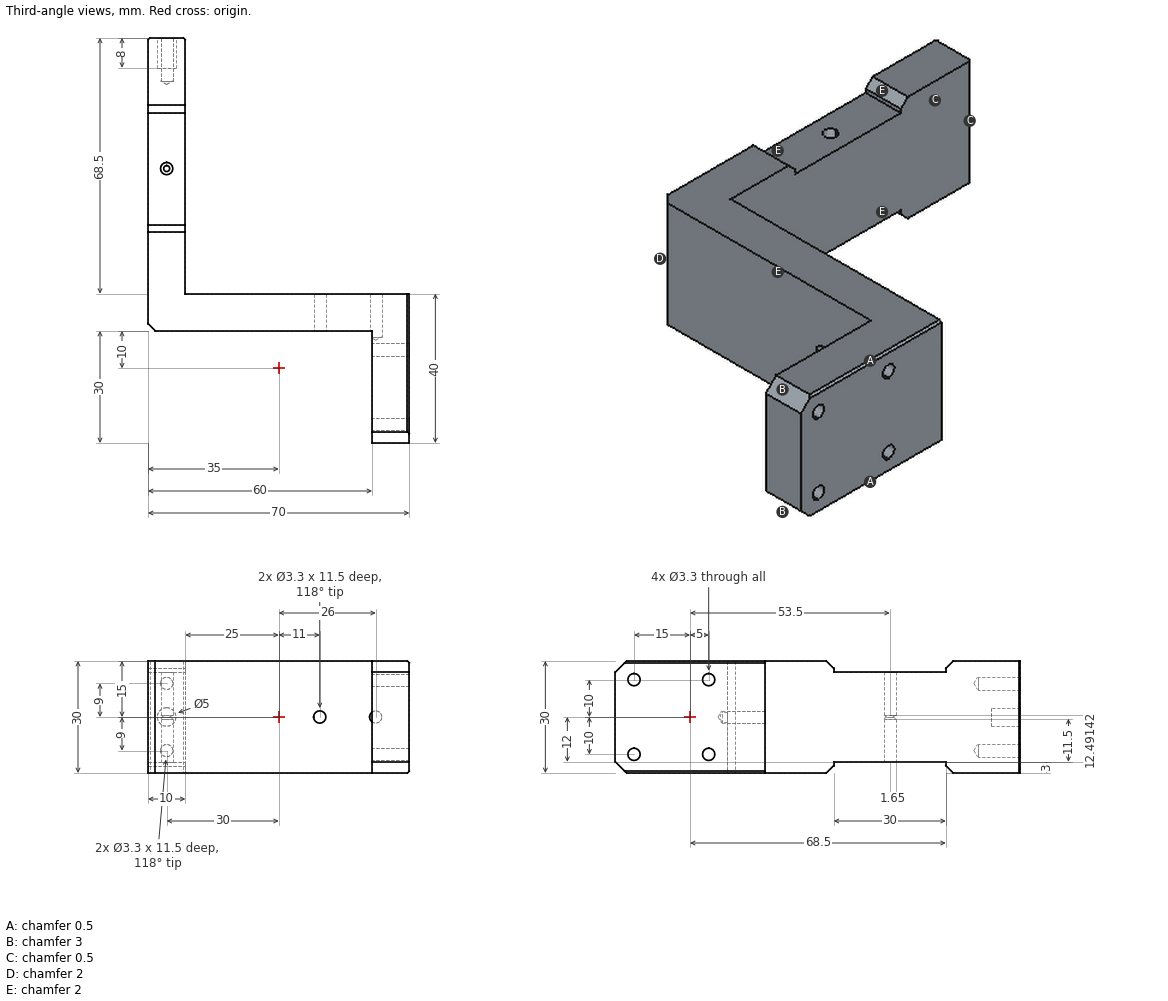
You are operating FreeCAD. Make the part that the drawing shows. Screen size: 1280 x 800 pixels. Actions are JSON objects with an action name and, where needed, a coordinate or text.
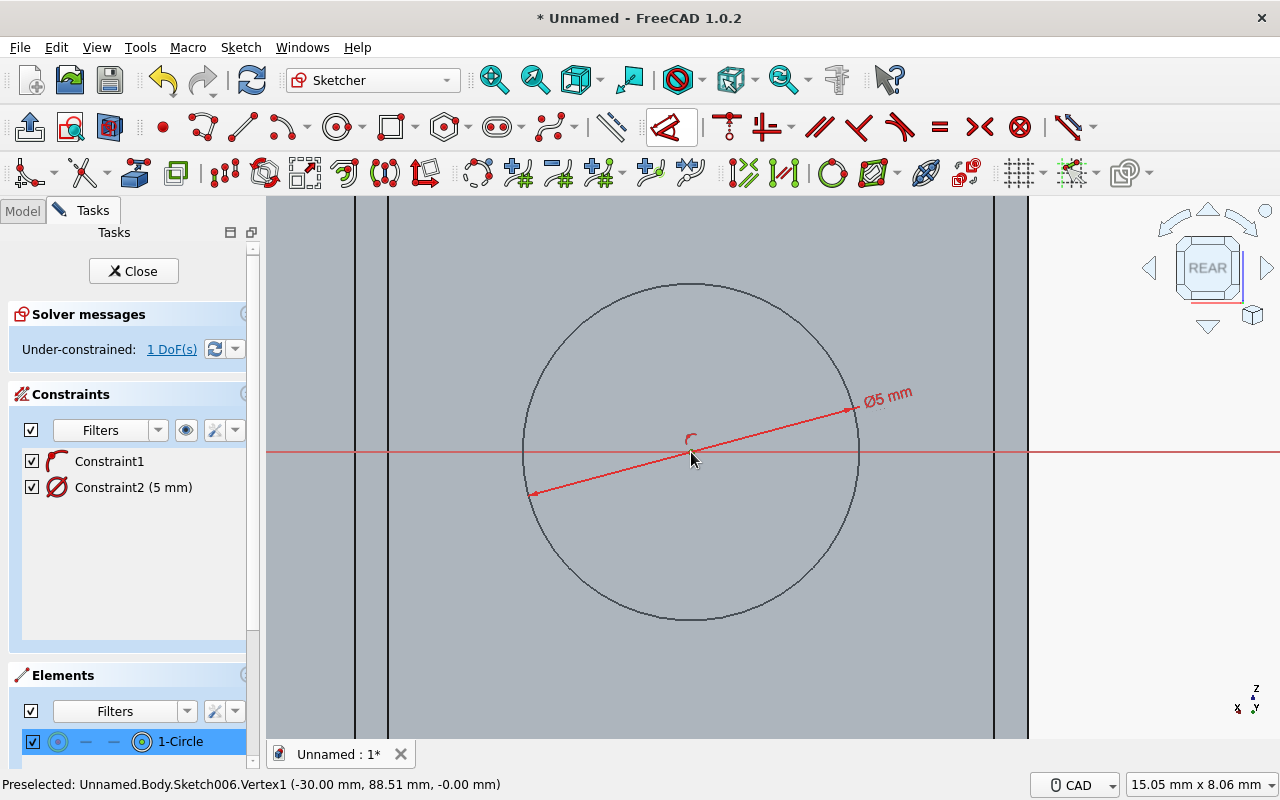
{"action": "left_click", "coordinate": [692, 128]}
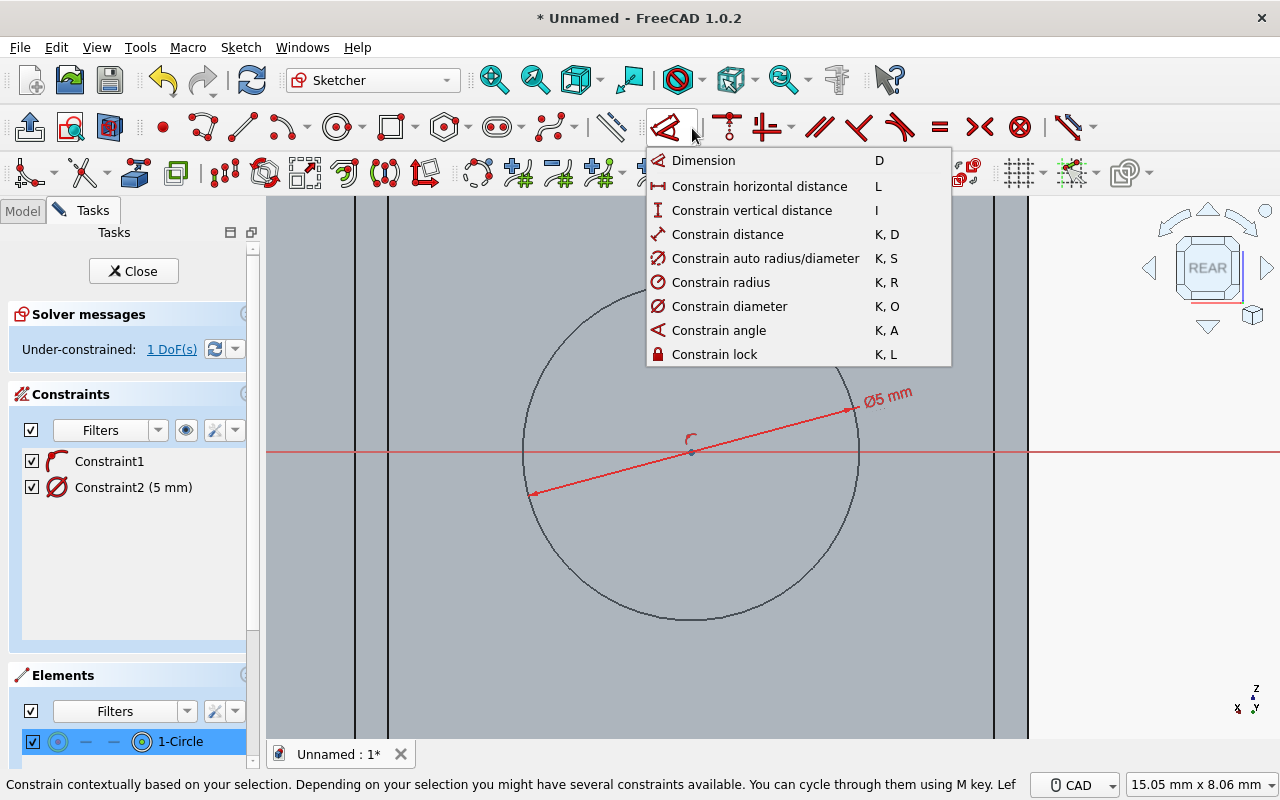
{"action": "left_click", "coordinate": [799, 186]}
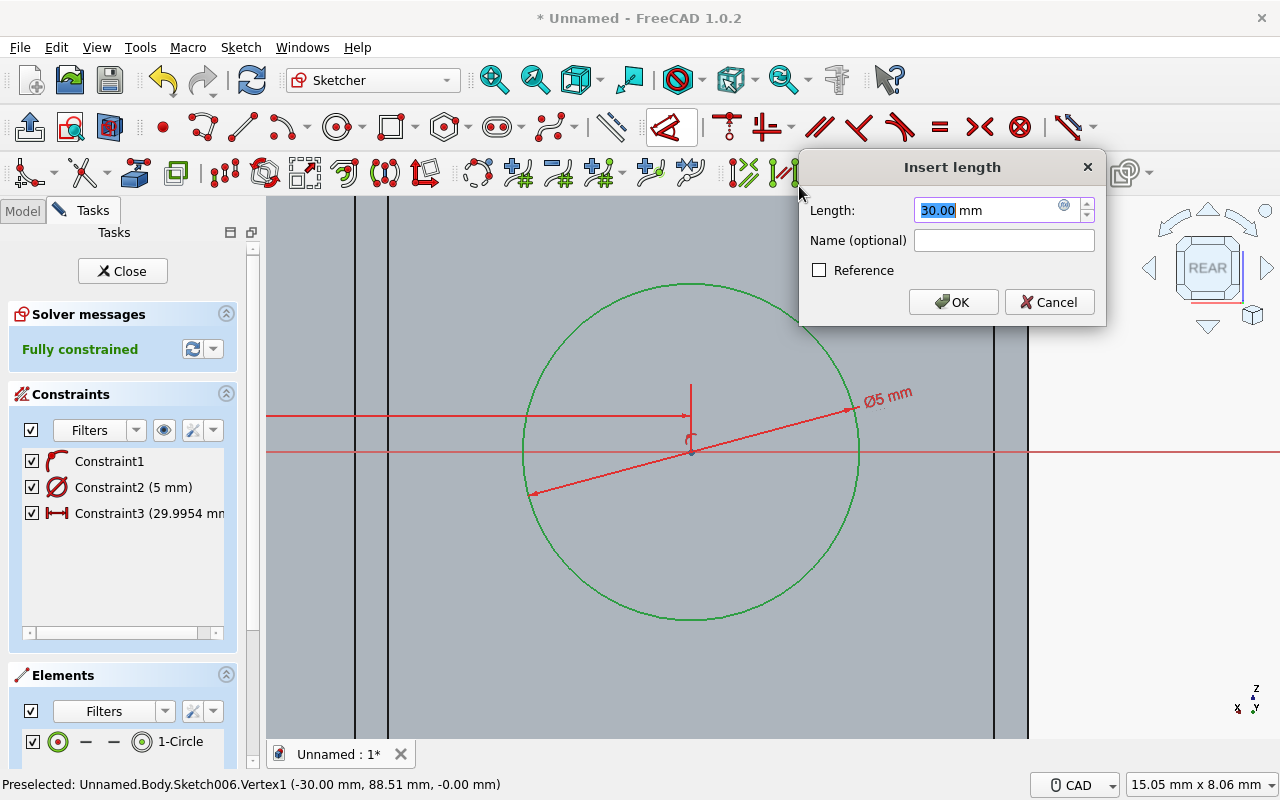
{"action": "type", "text": "30"}
{"action": "key", "text": "Return"}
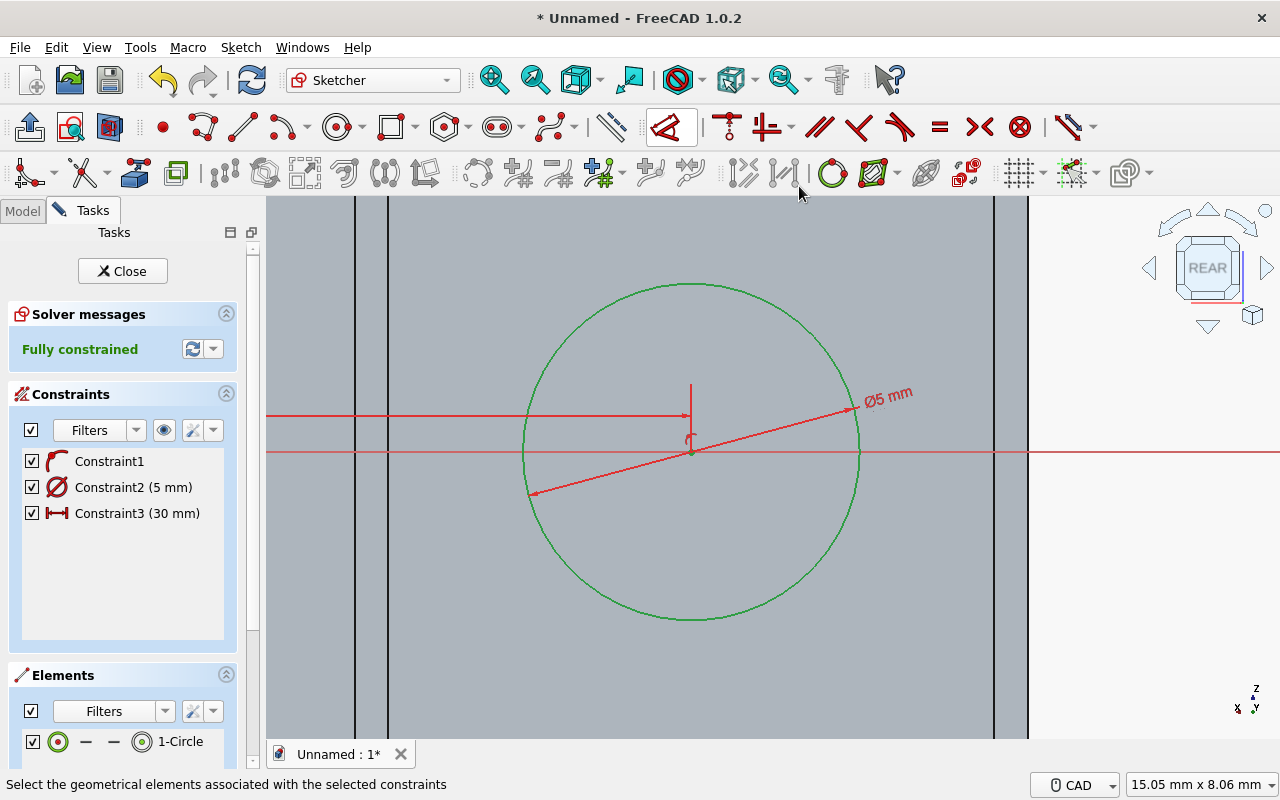
{"action": "left_click", "coordinate": [123, 271]}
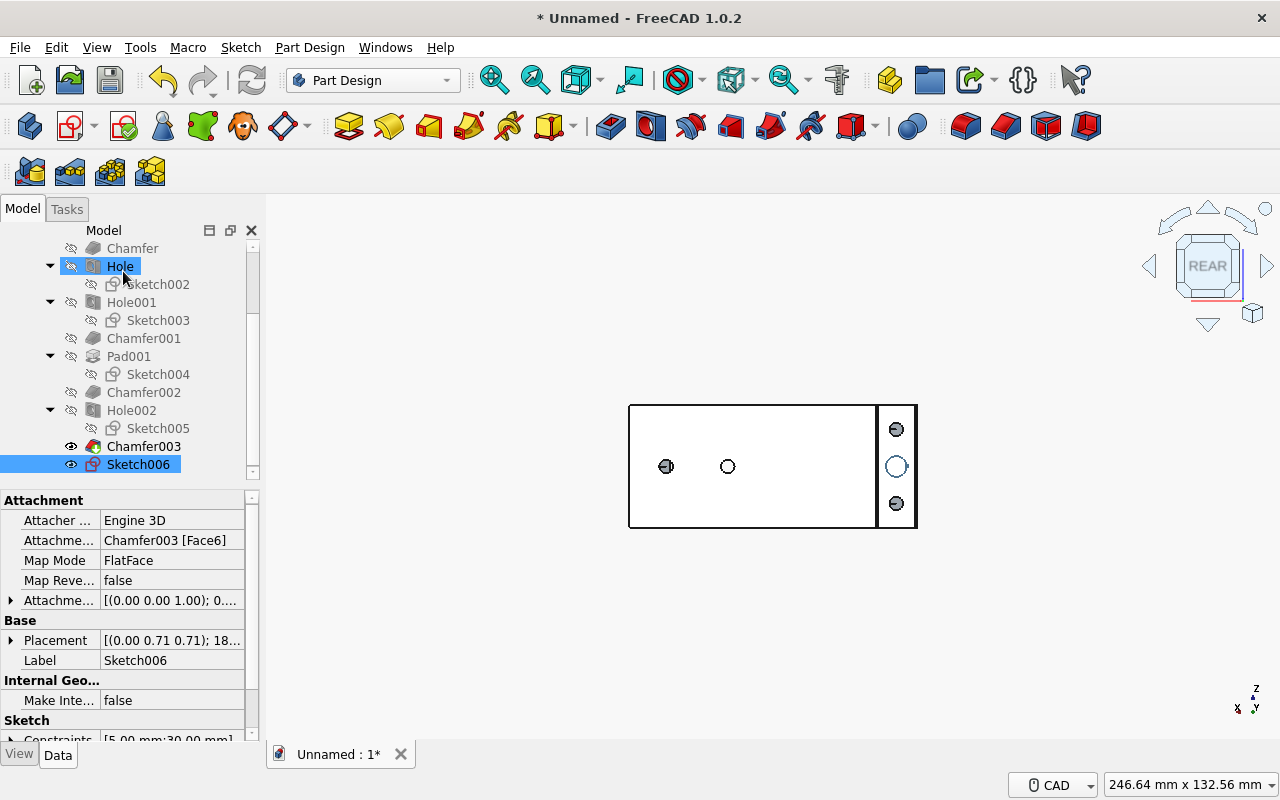
{"action": "left_click", "coordinate": [612, 126]}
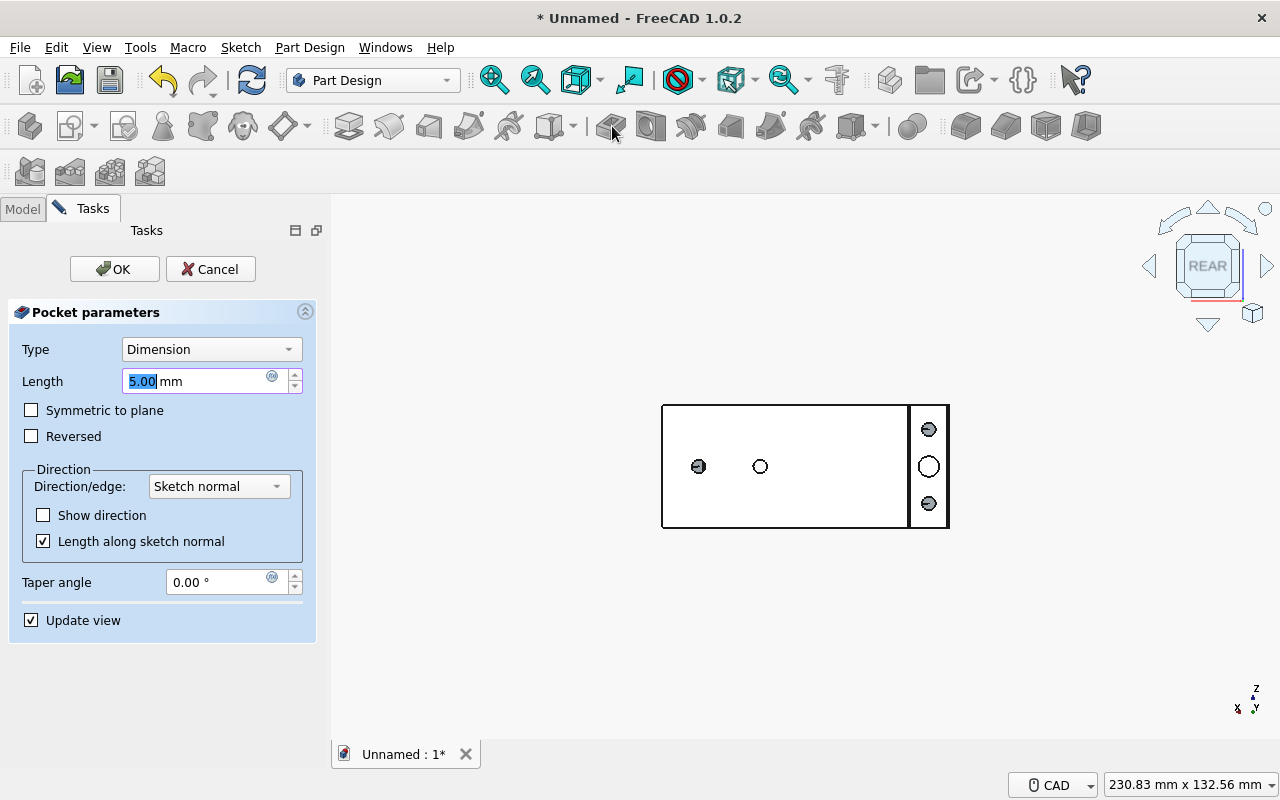
{"action": "type", "text": "8"}
{"action": "key", "text": "Tab"}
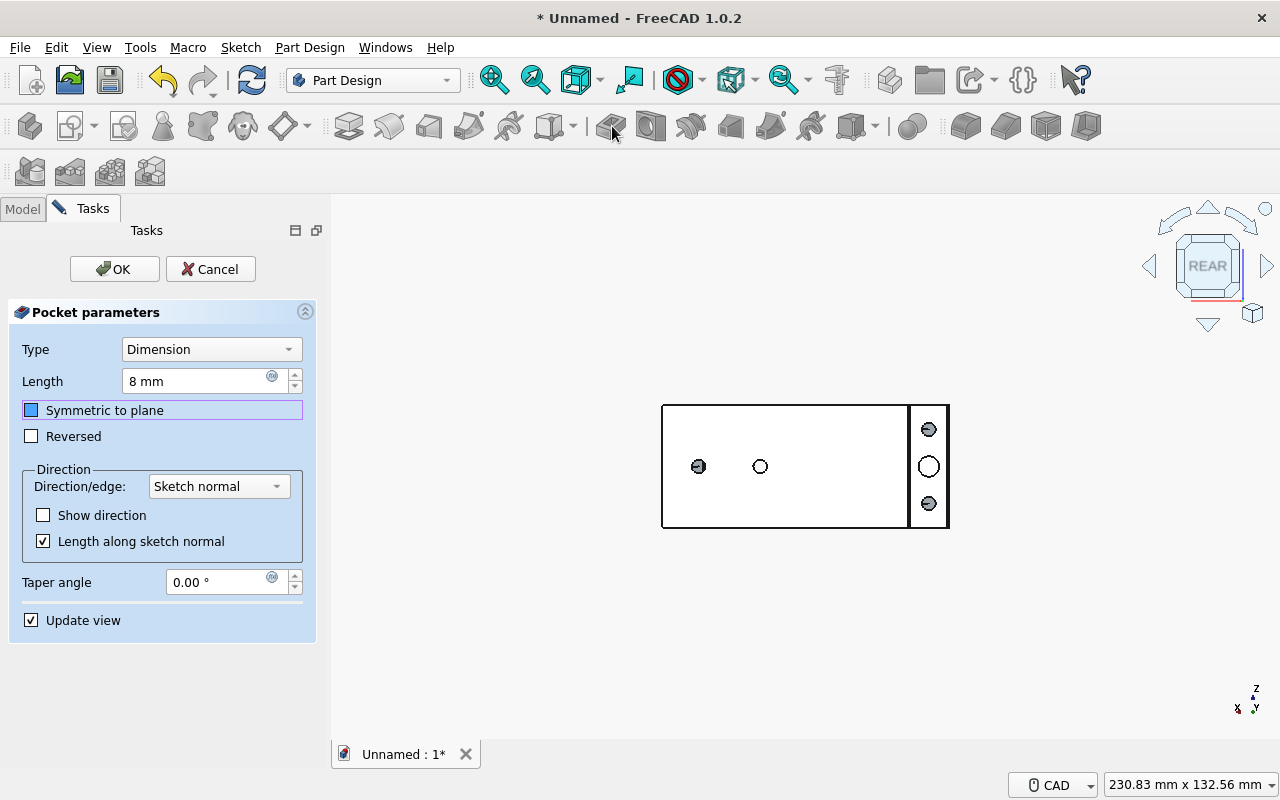
{"action": "left_click", "coordinate": [115, 269]}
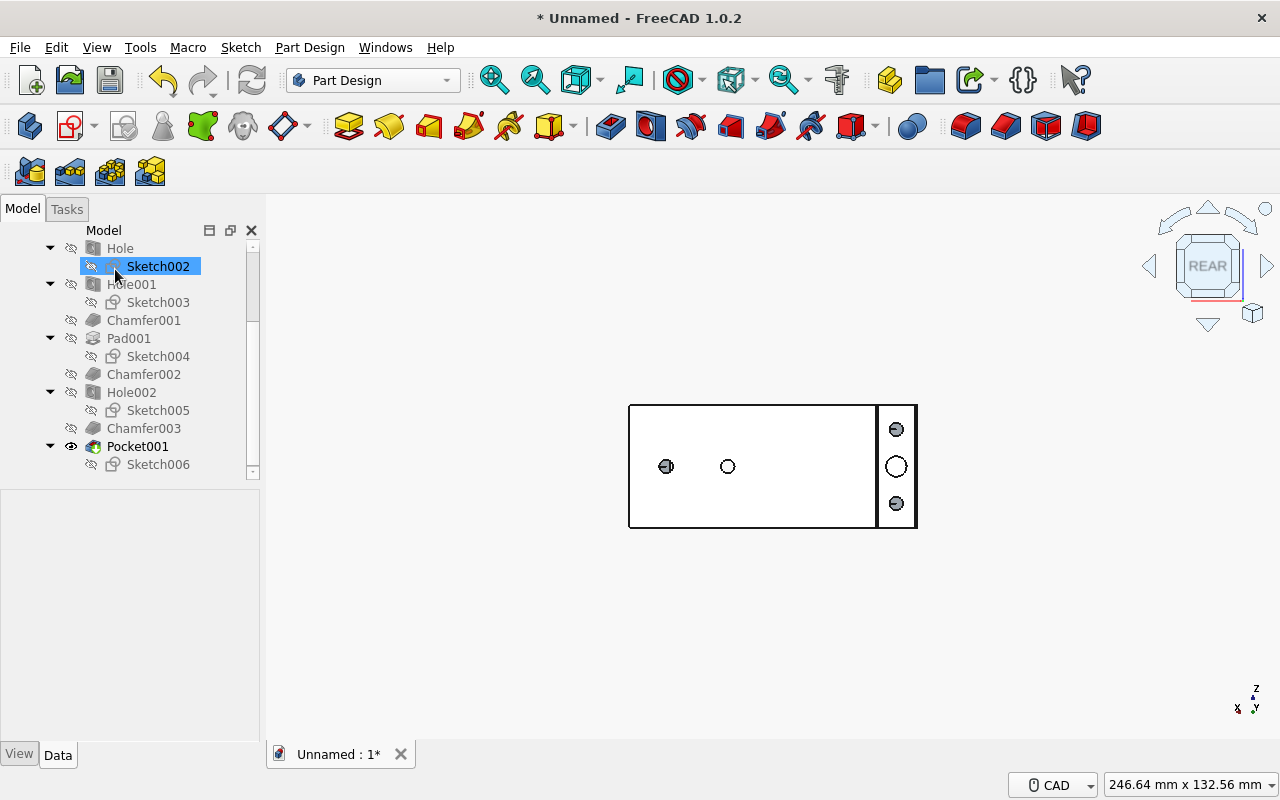
{"action": "left_click", "coordinate": [496, 80]}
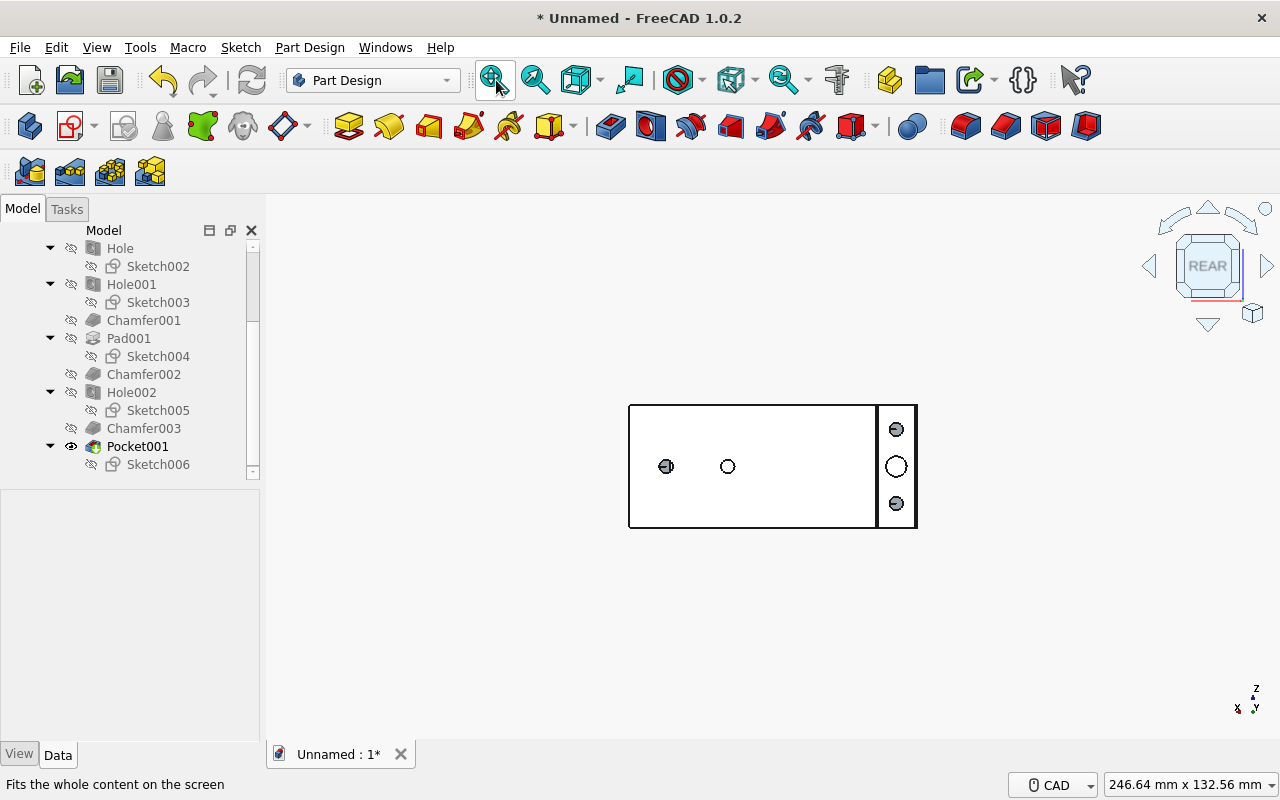
{"action": "key", "text": "6"}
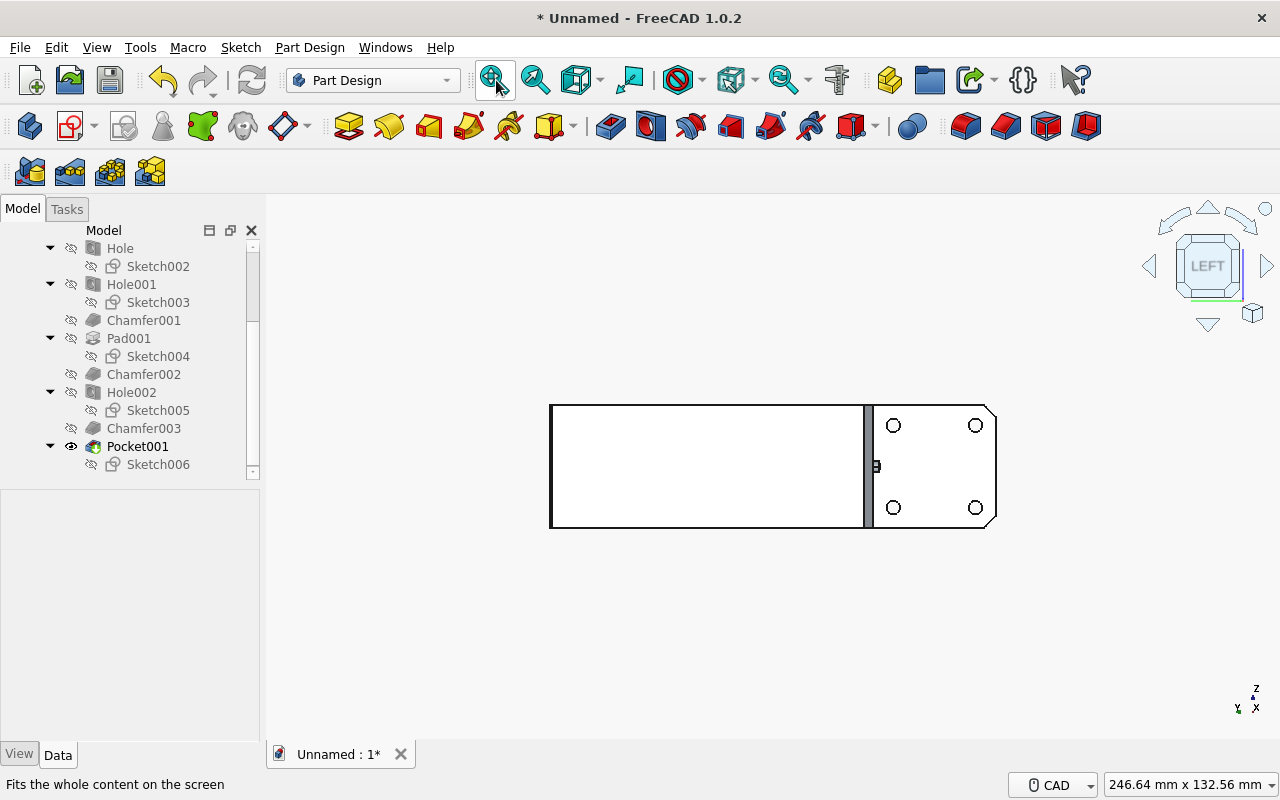
{"action": "left_click", "coordinate": [496, 80]}